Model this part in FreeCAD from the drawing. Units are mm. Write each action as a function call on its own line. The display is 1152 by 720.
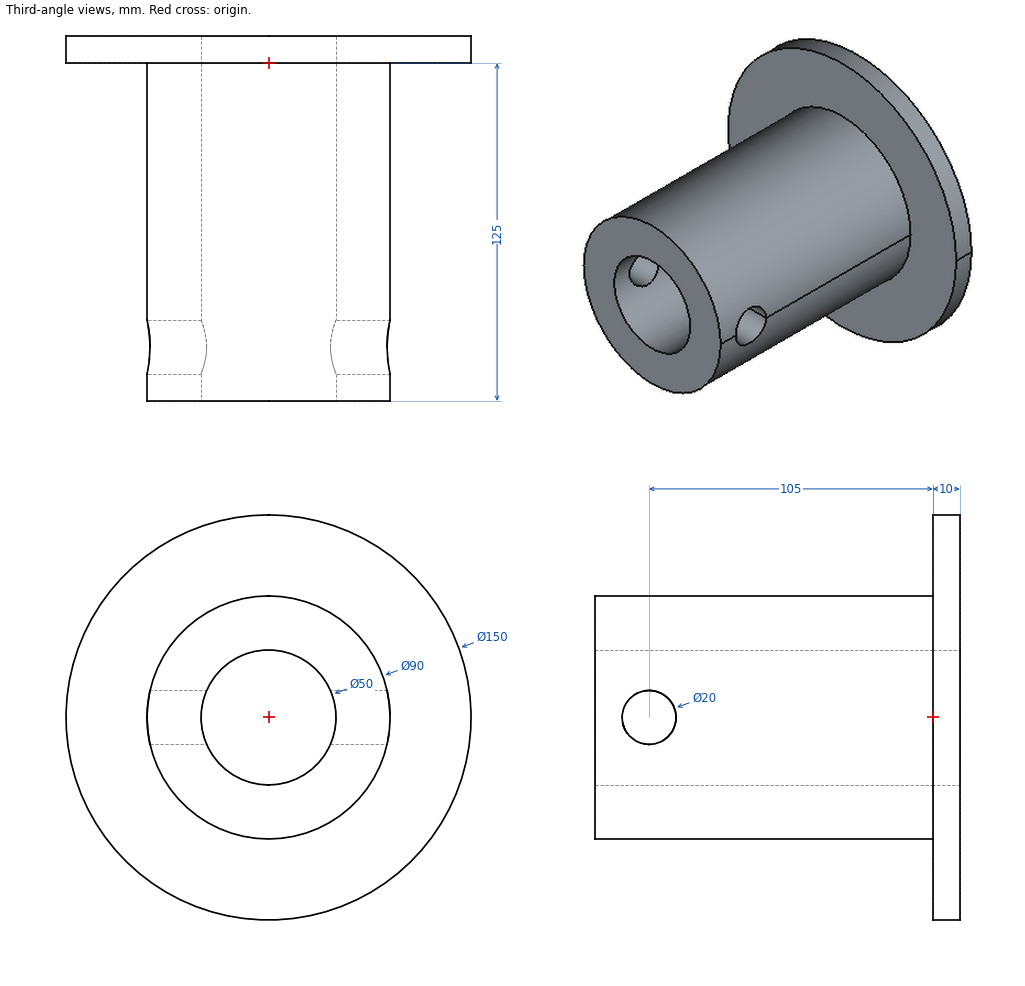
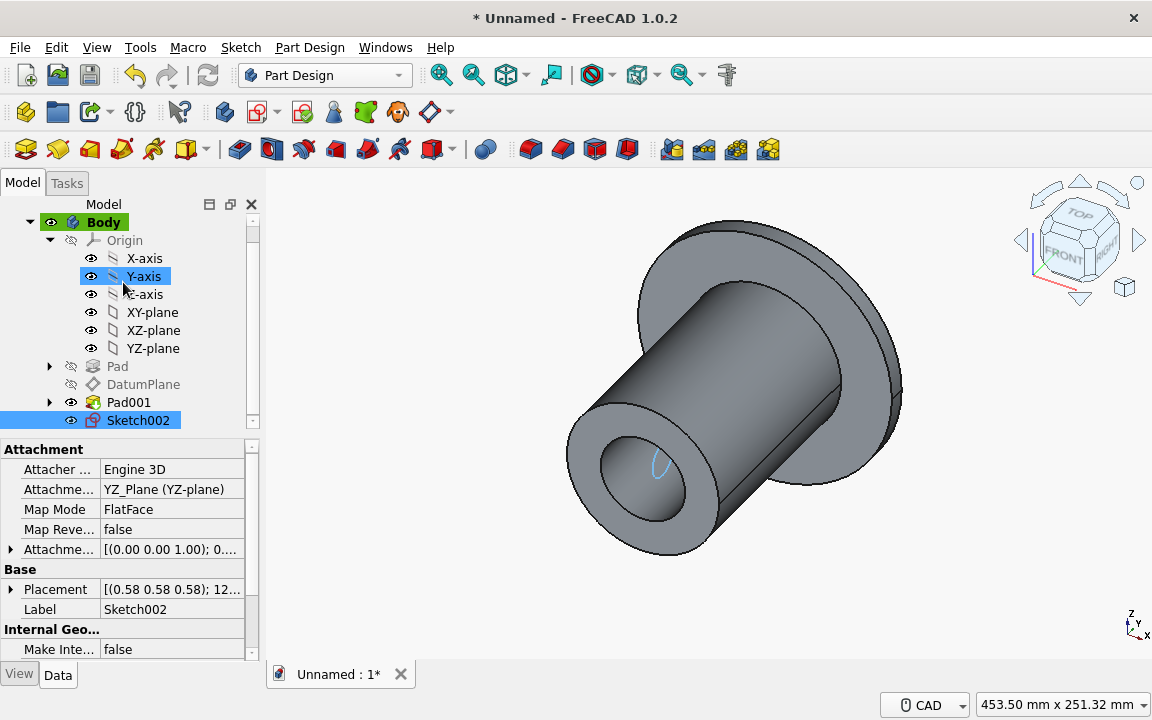
click(240, 150)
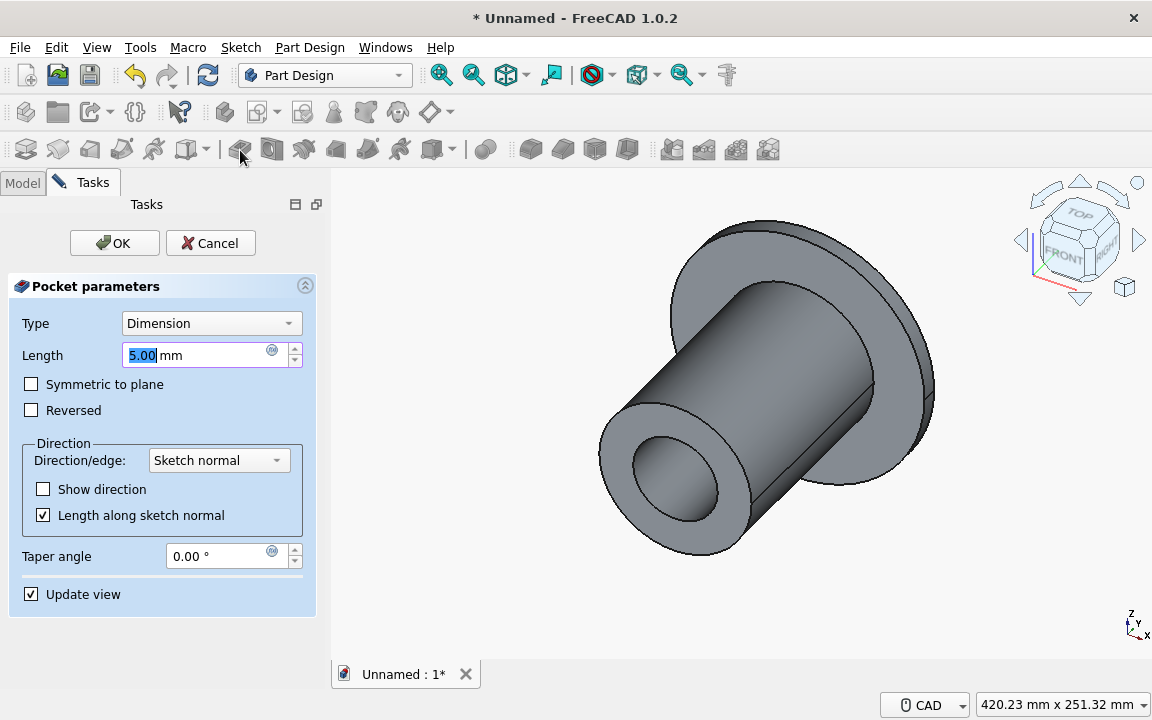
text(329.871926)
key(Tab)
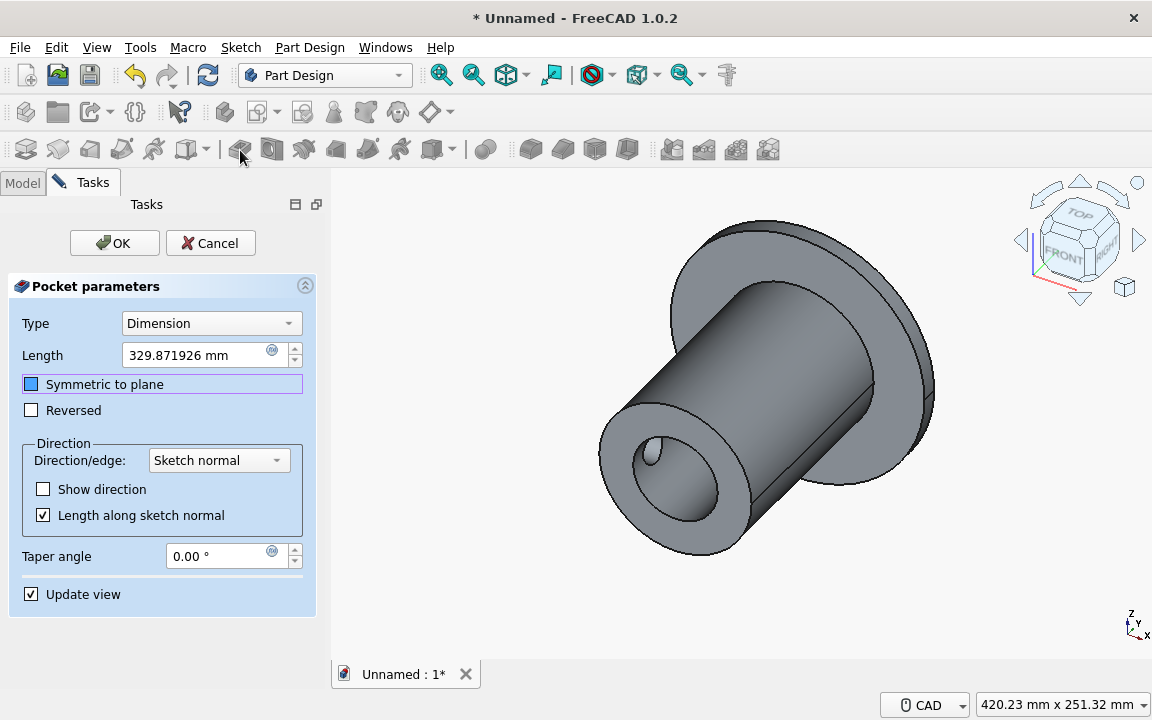
click(30, 384)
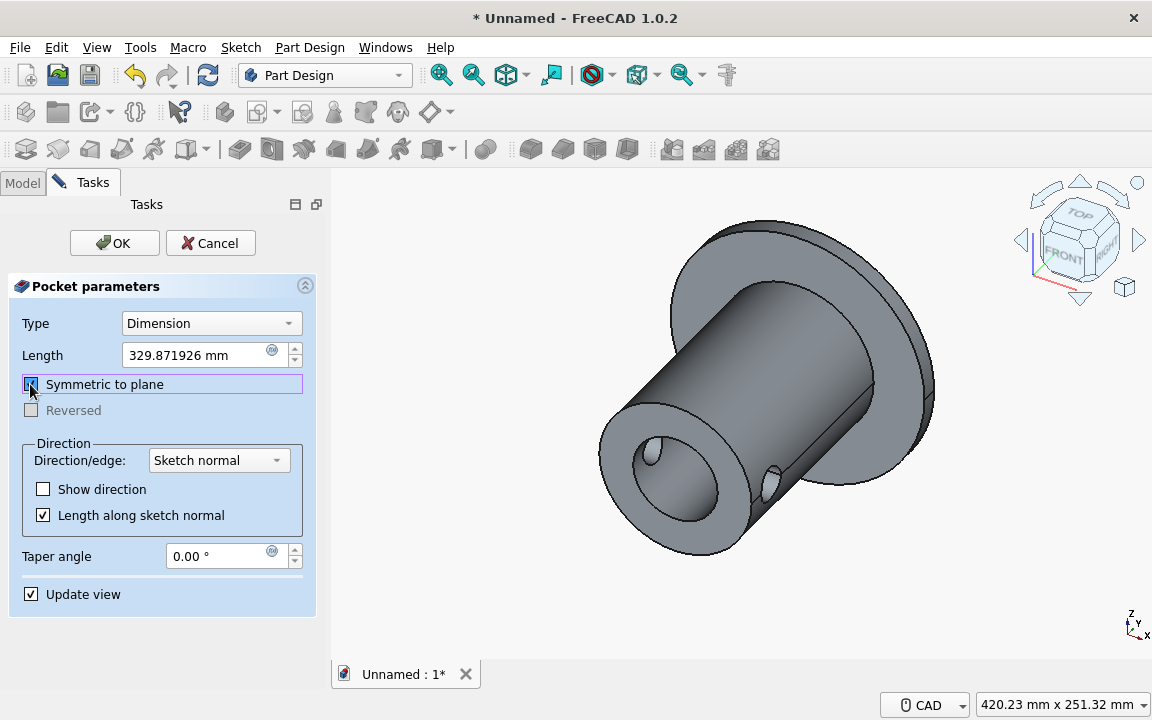
click(115, 243)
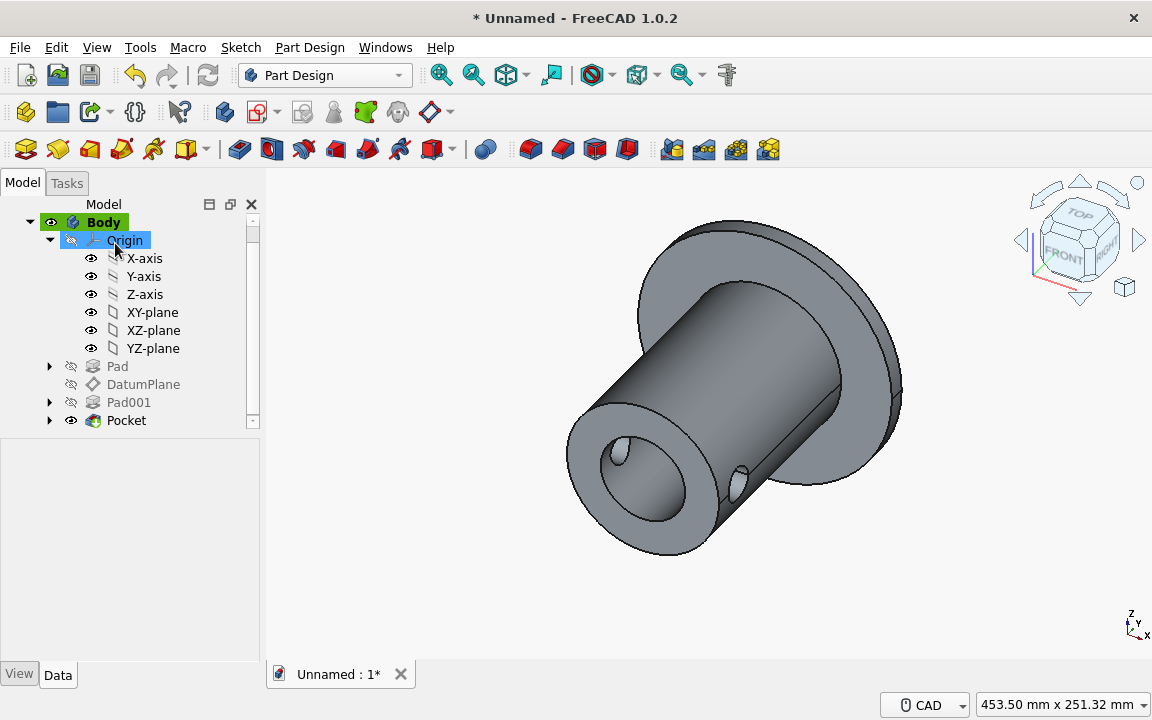
key(0)